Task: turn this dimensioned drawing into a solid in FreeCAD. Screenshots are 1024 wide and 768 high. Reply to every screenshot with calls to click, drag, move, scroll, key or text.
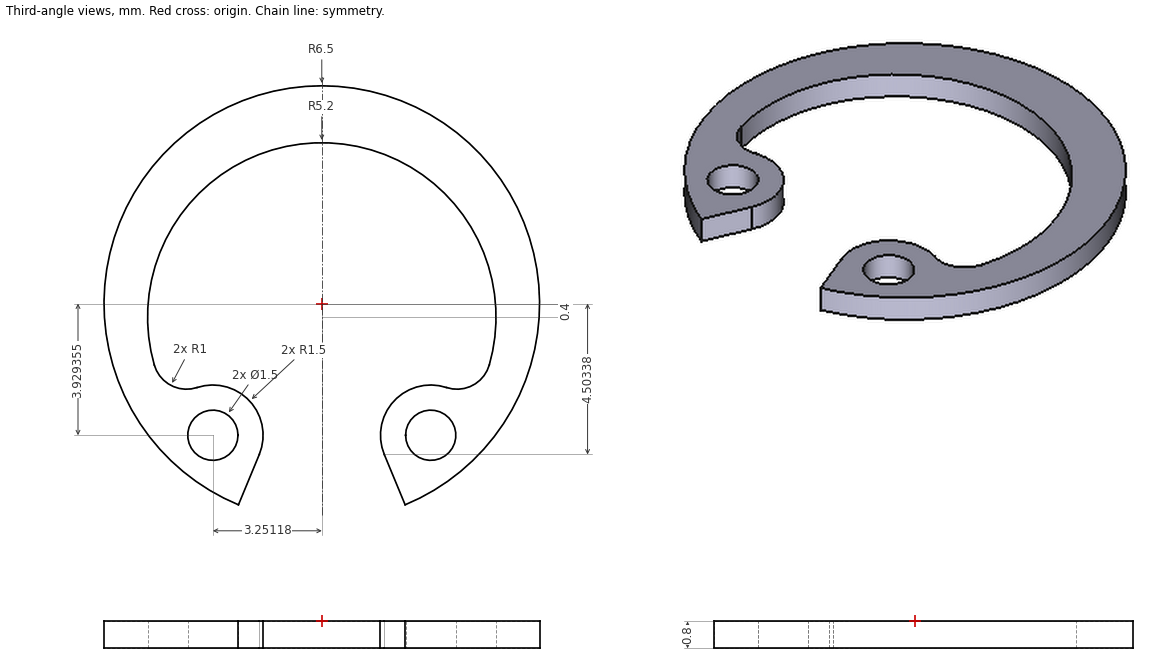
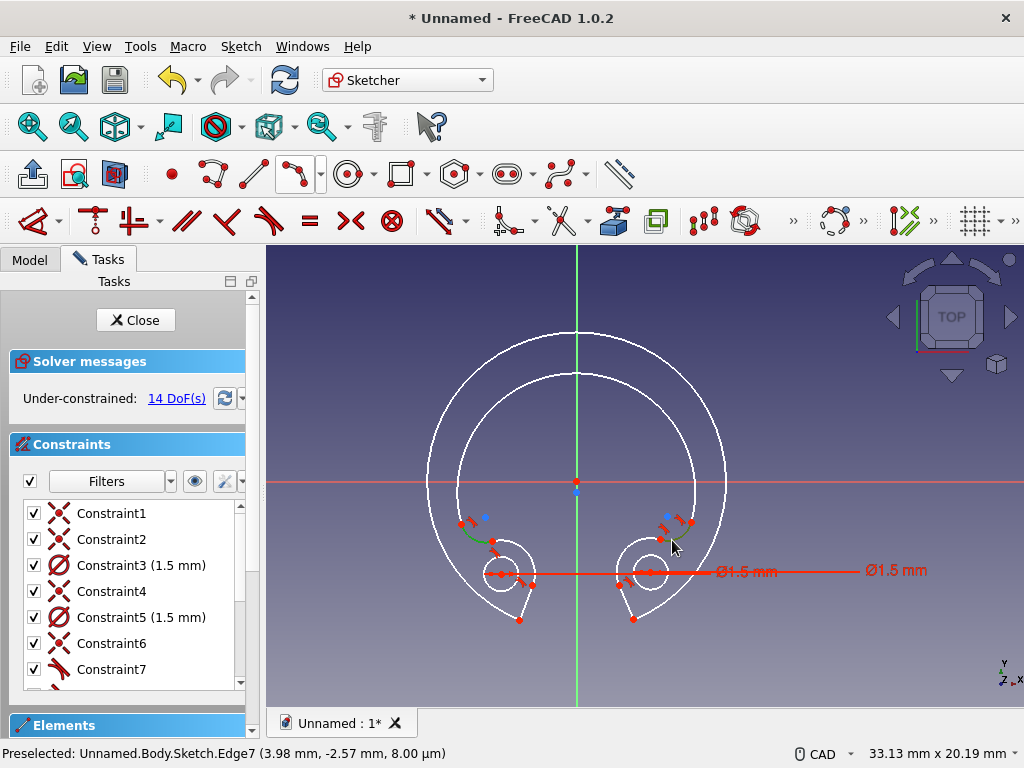
key(e)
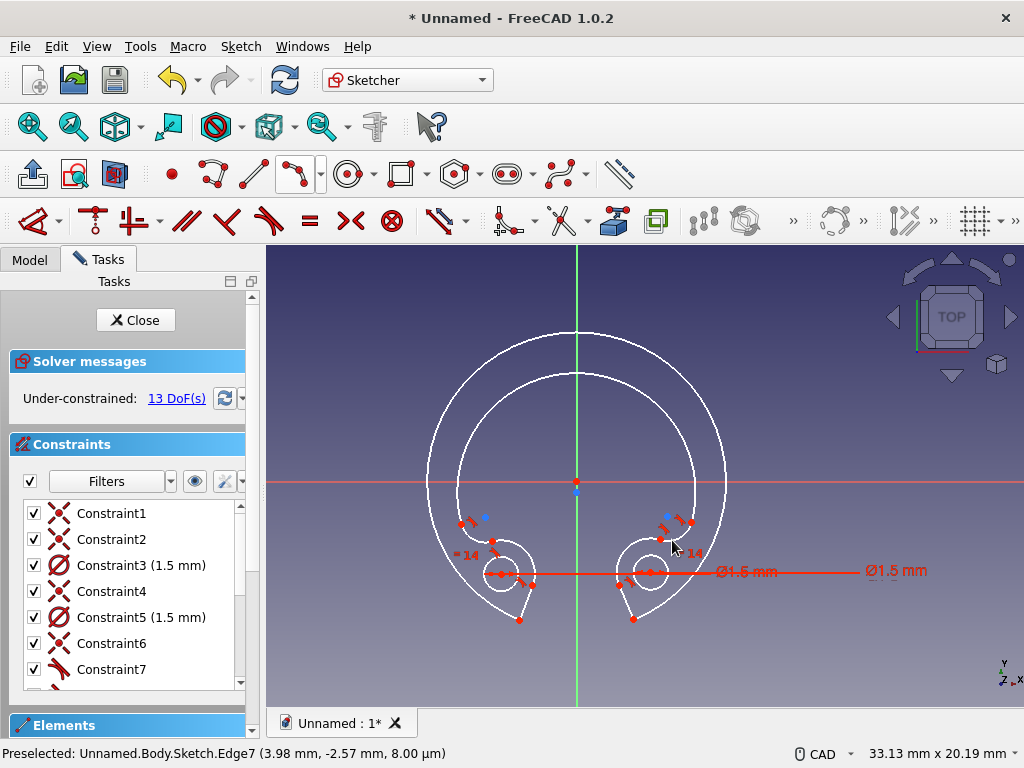
click(533, 564)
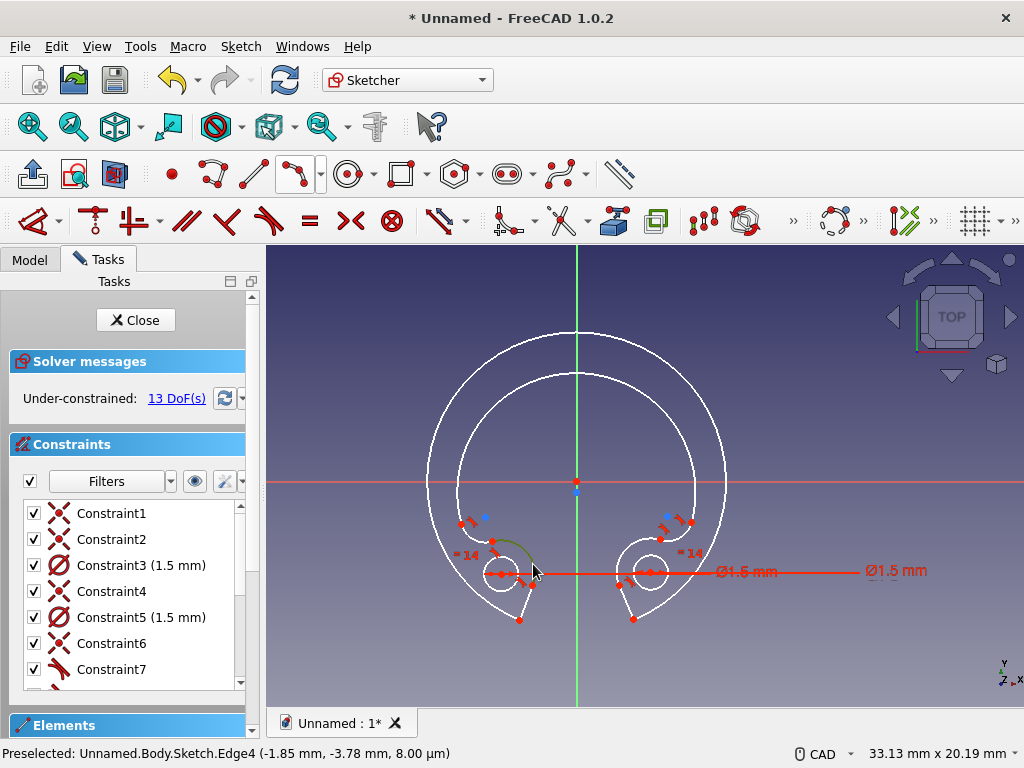
click(638, 541)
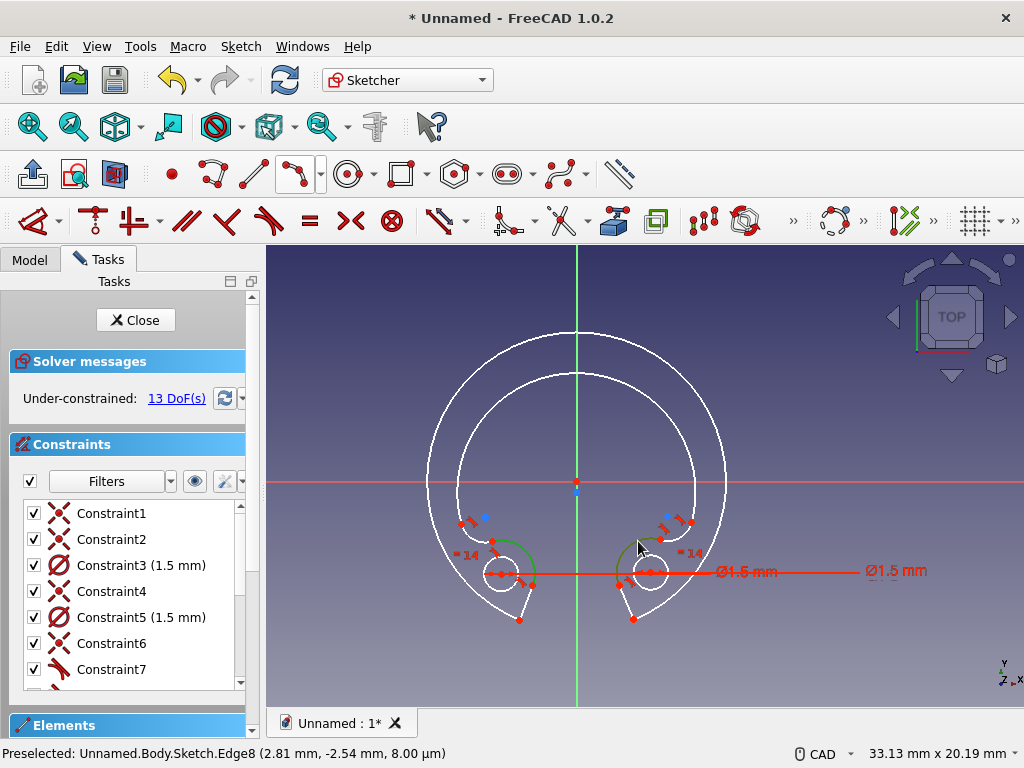
key(e)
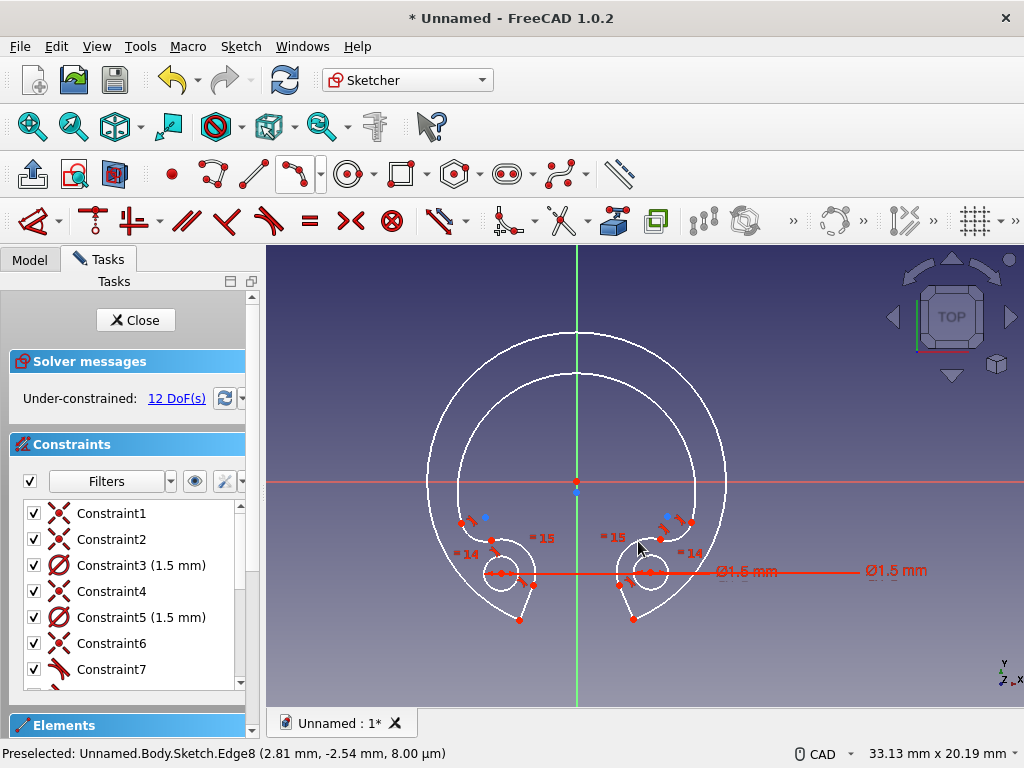
click(577, 492)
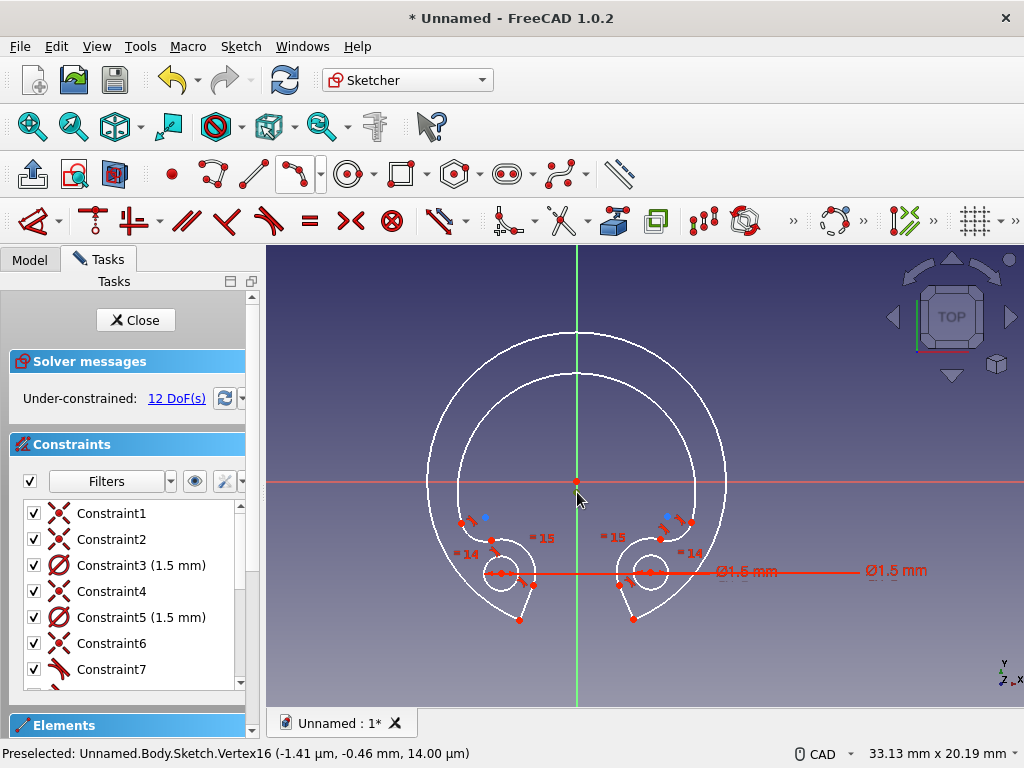
click(577, 650)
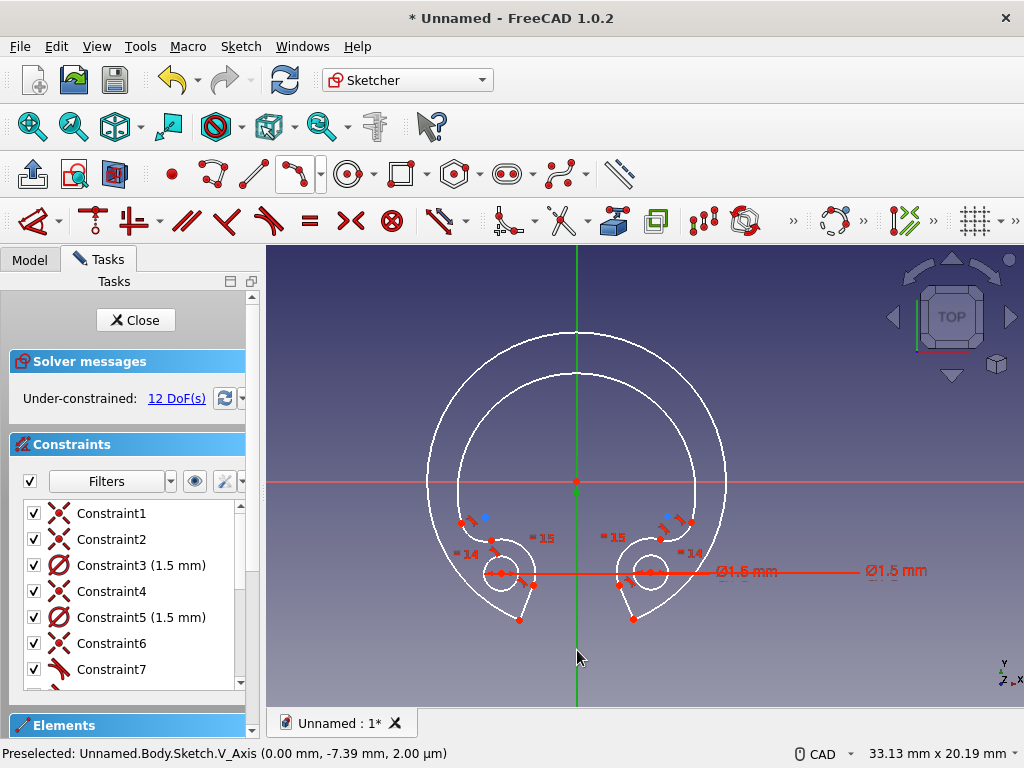
key(c)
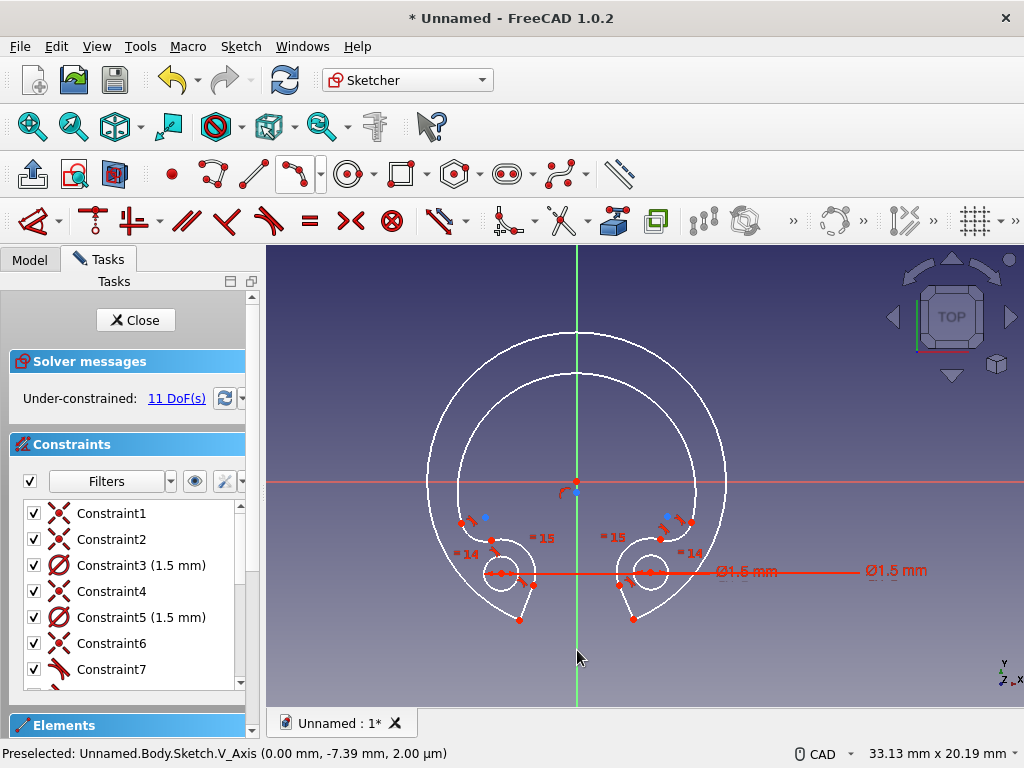
click(501, 574)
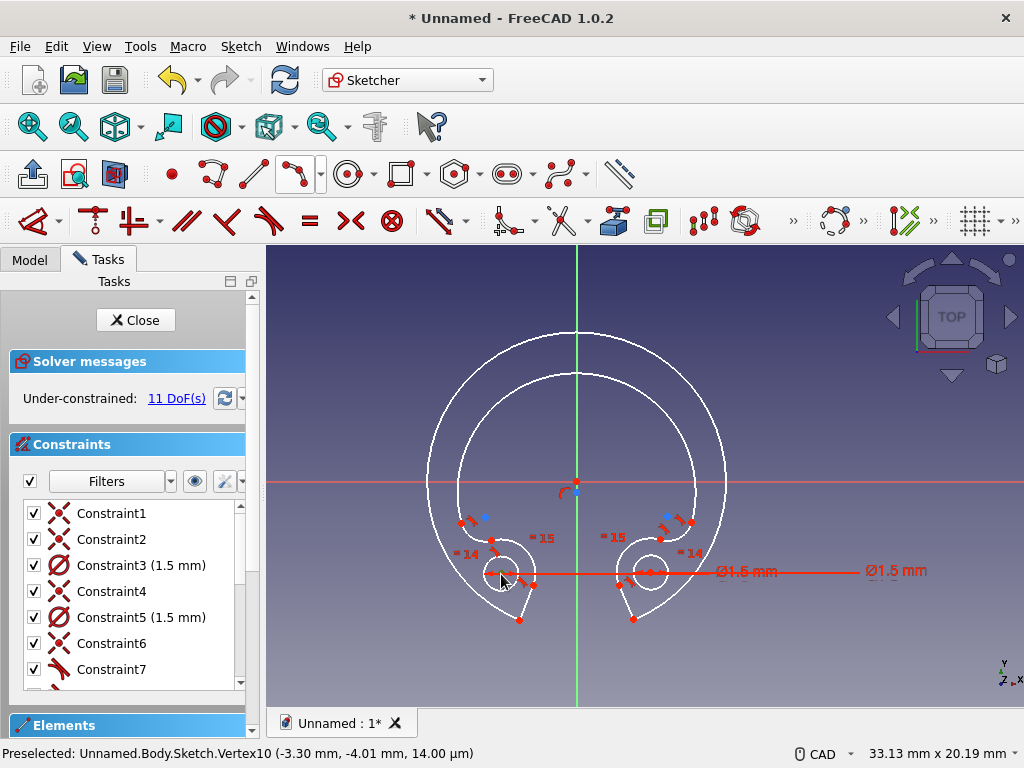
click(651, 572)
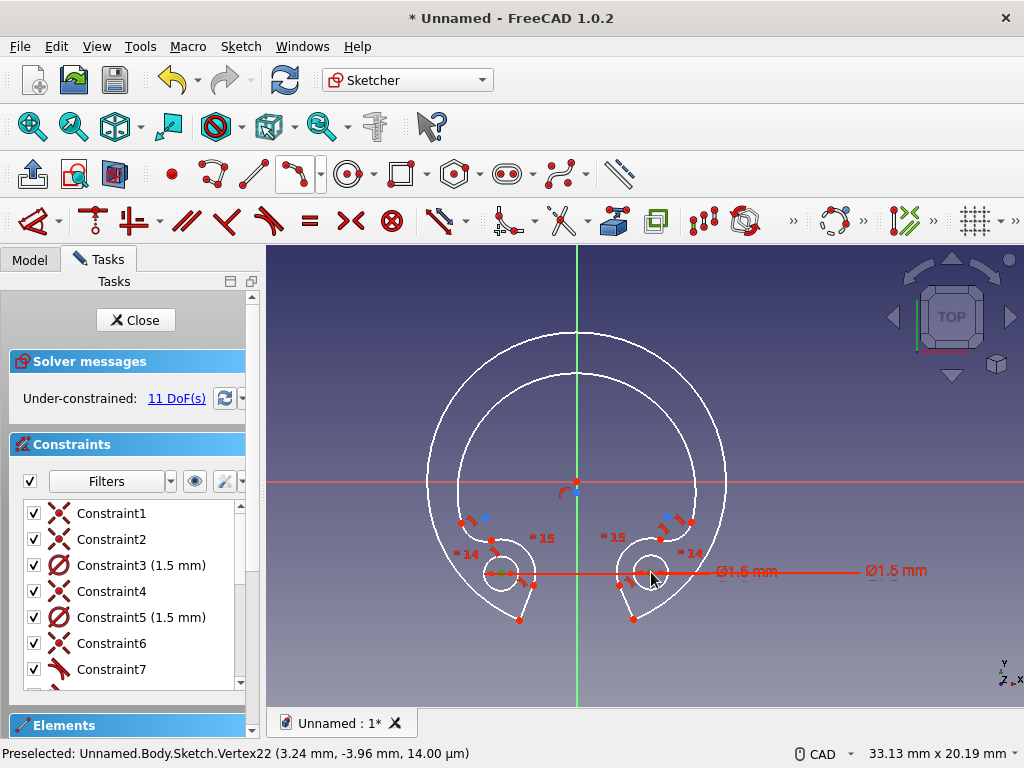
click(577, 650)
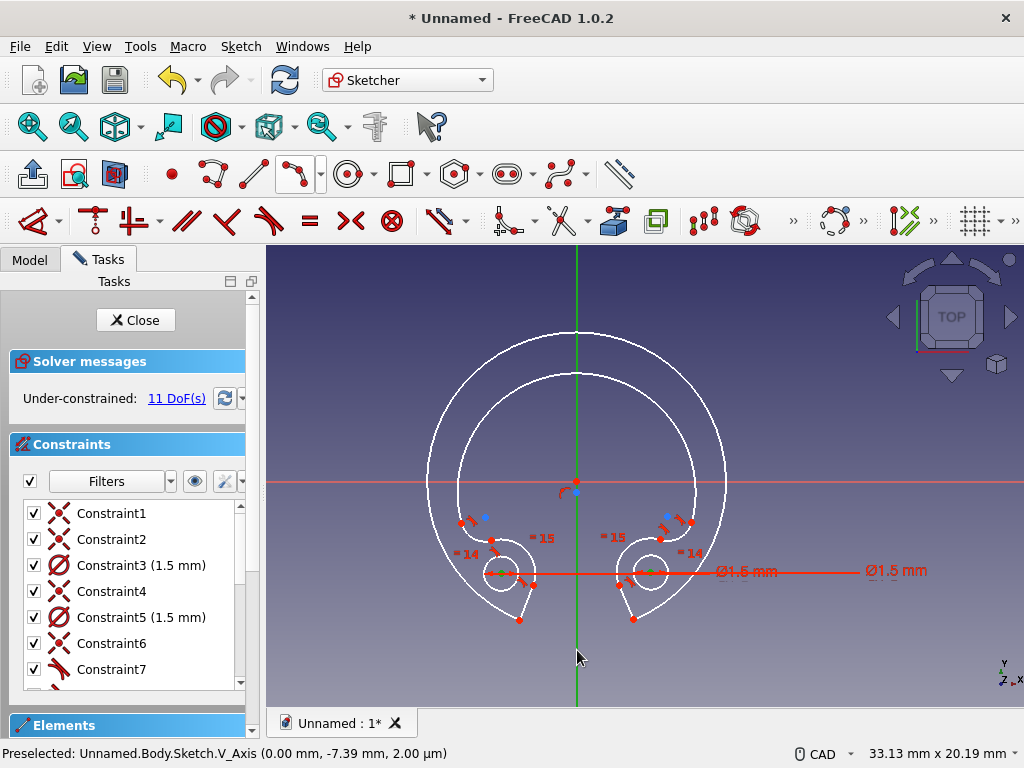
key(s)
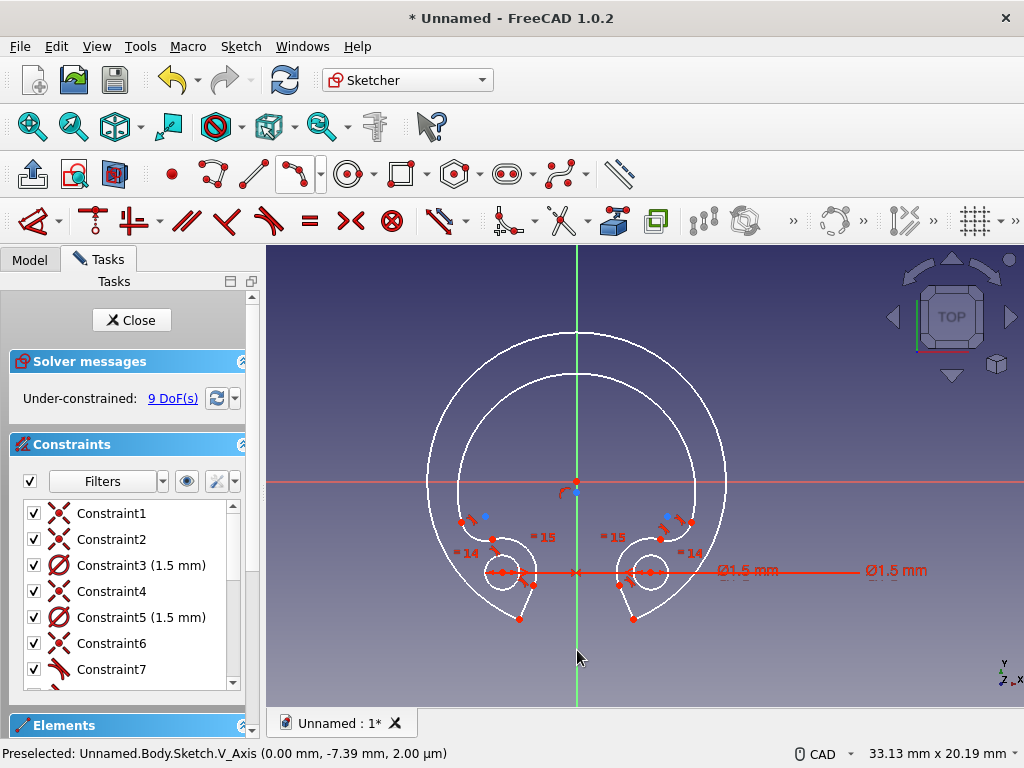
key(d)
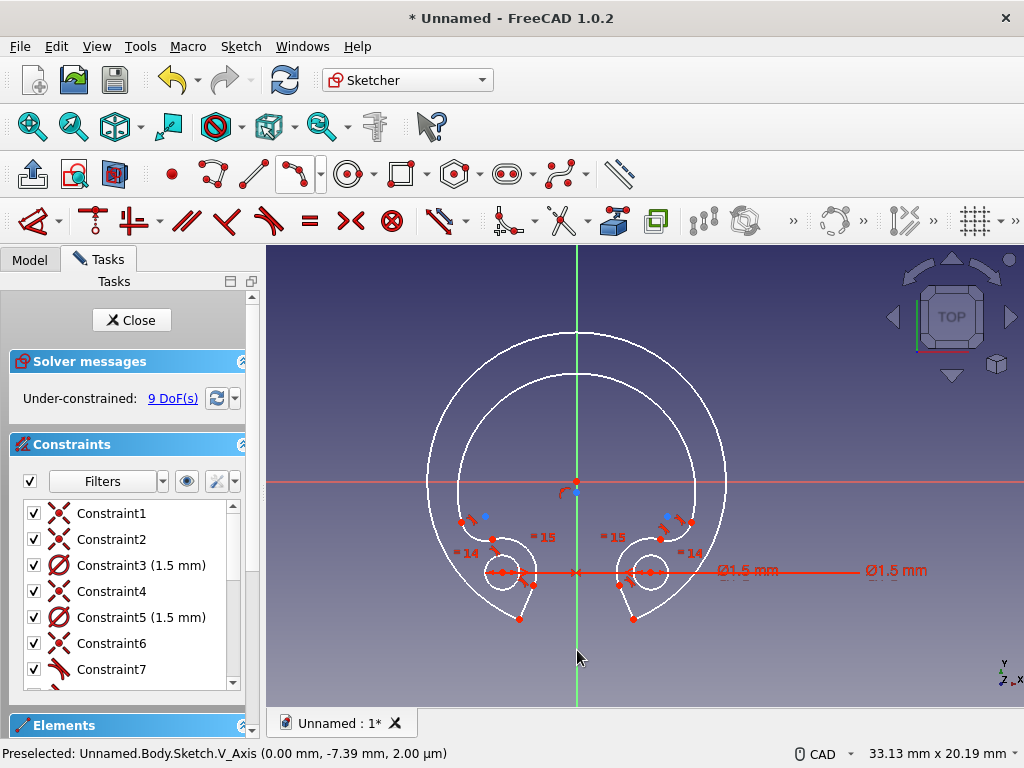
click(710, 414)
click(739, 399)